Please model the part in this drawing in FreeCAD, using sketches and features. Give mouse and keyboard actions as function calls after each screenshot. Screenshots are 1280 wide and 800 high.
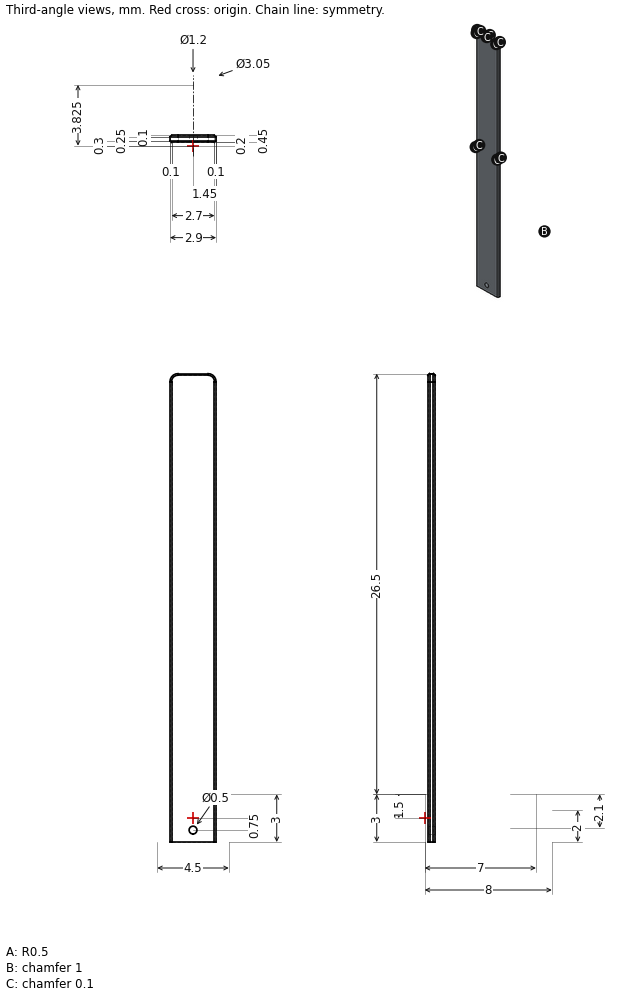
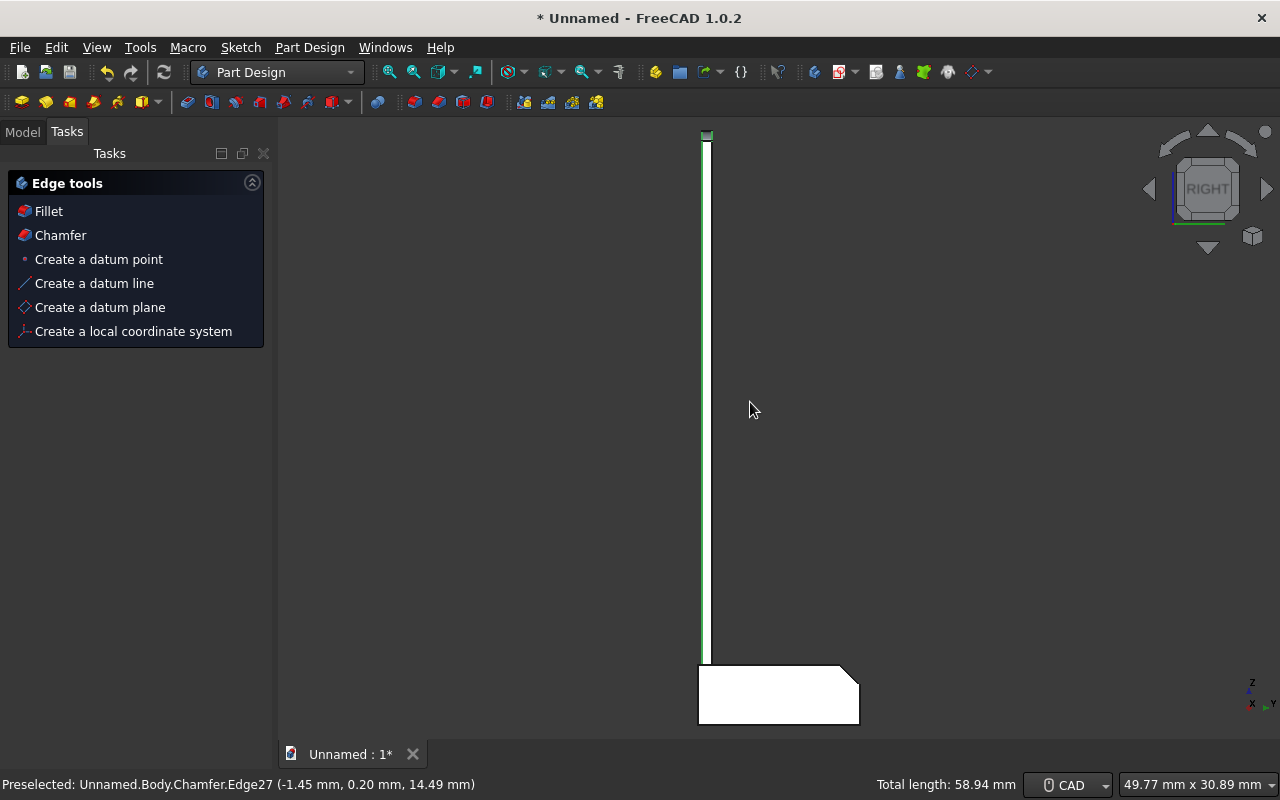
click(712, 402, ctrl)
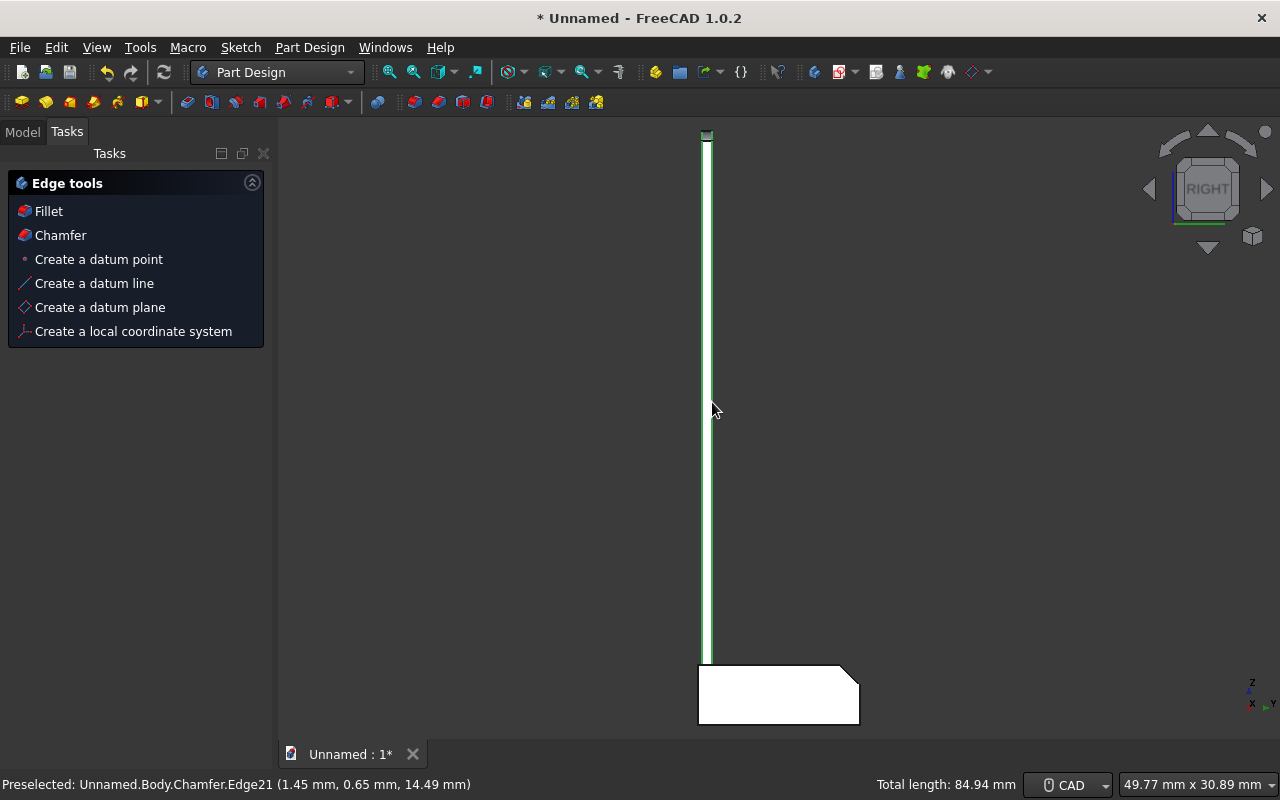
key(5)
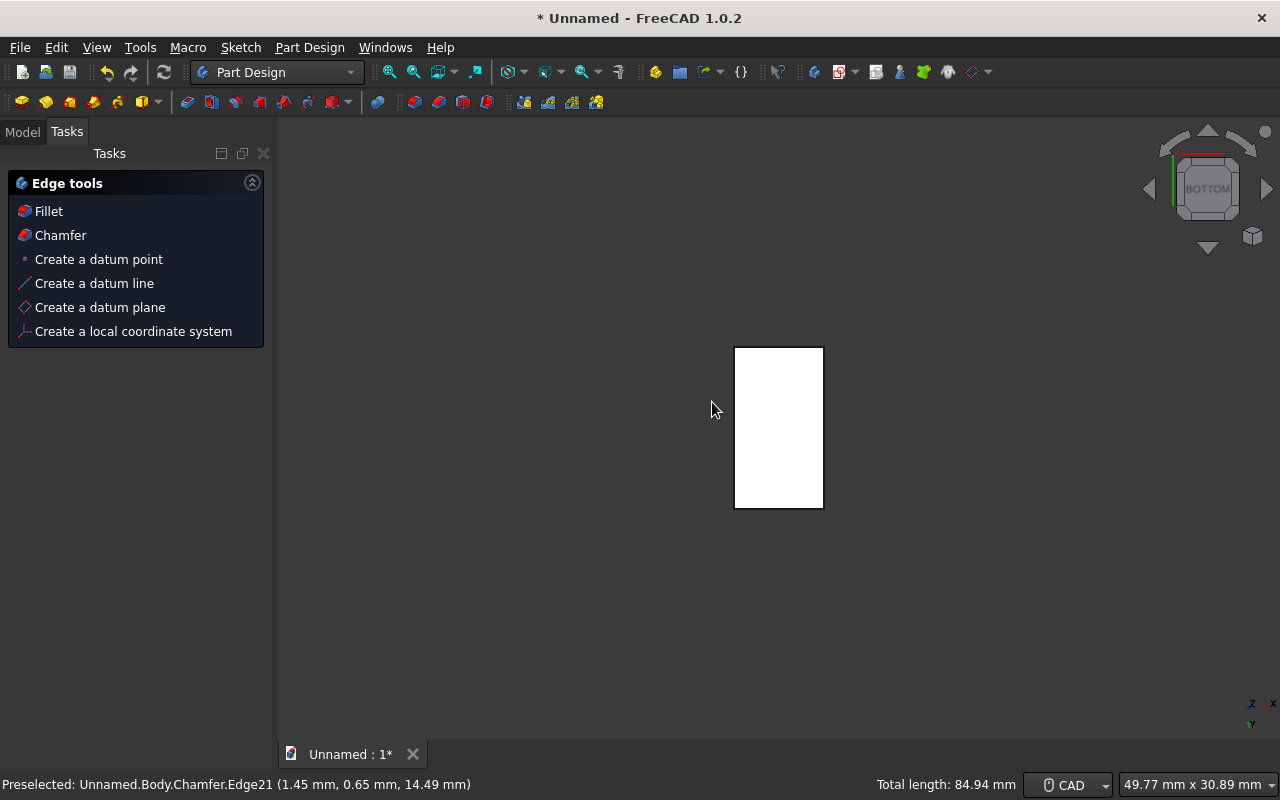
key(v)
key(f)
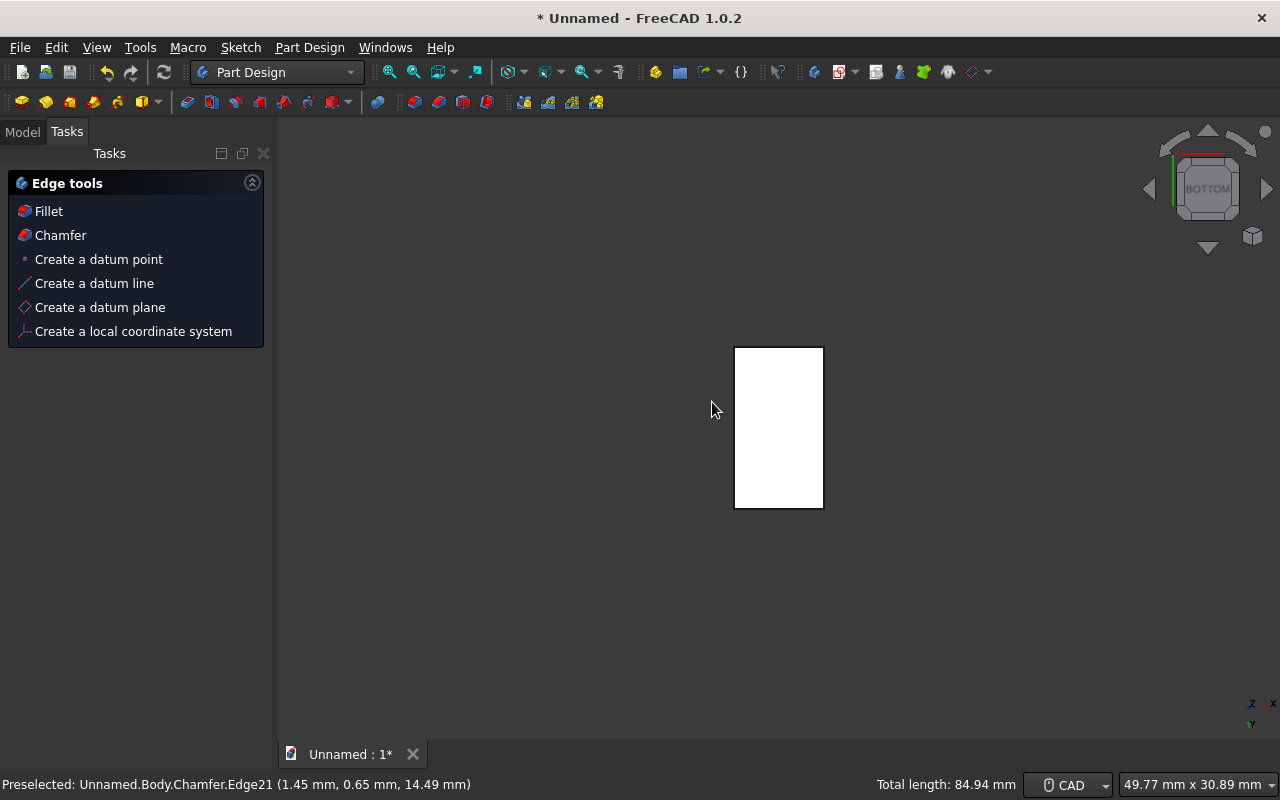
key(4)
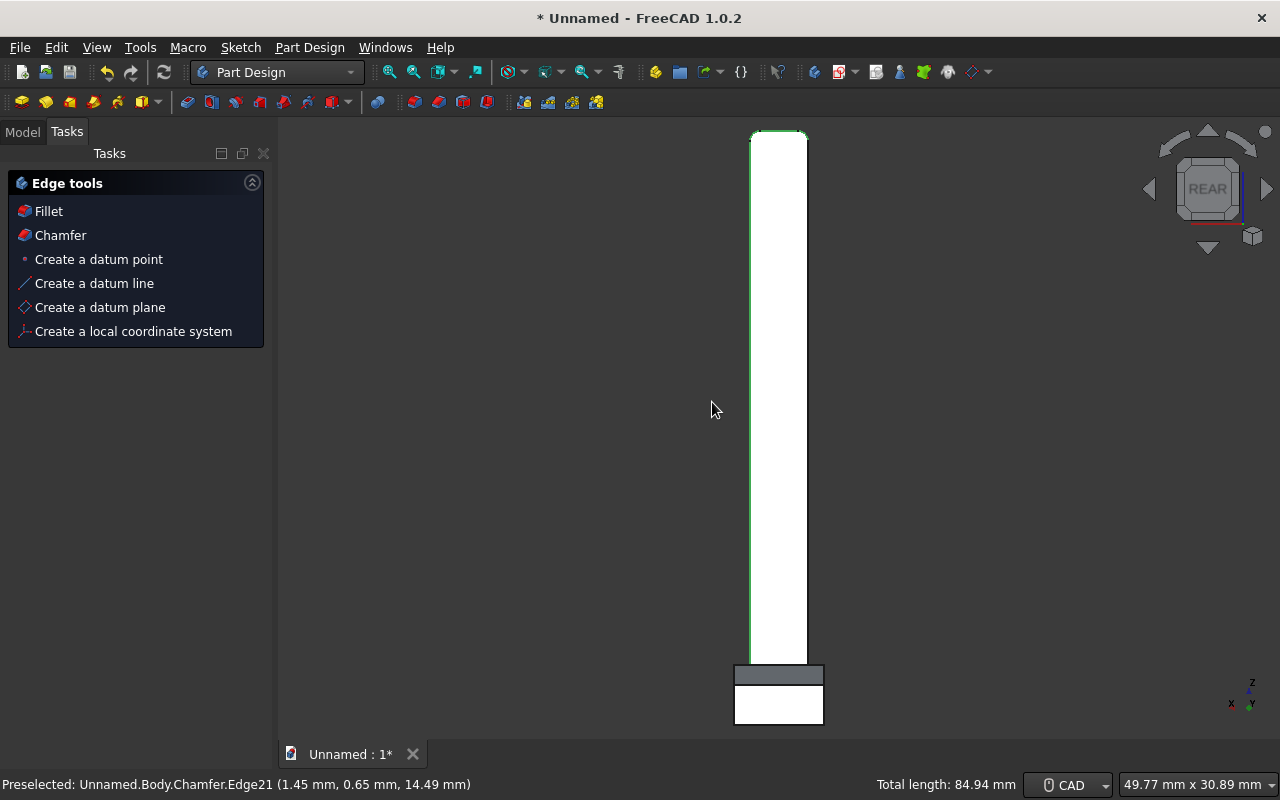
click(808, 402, ctrl)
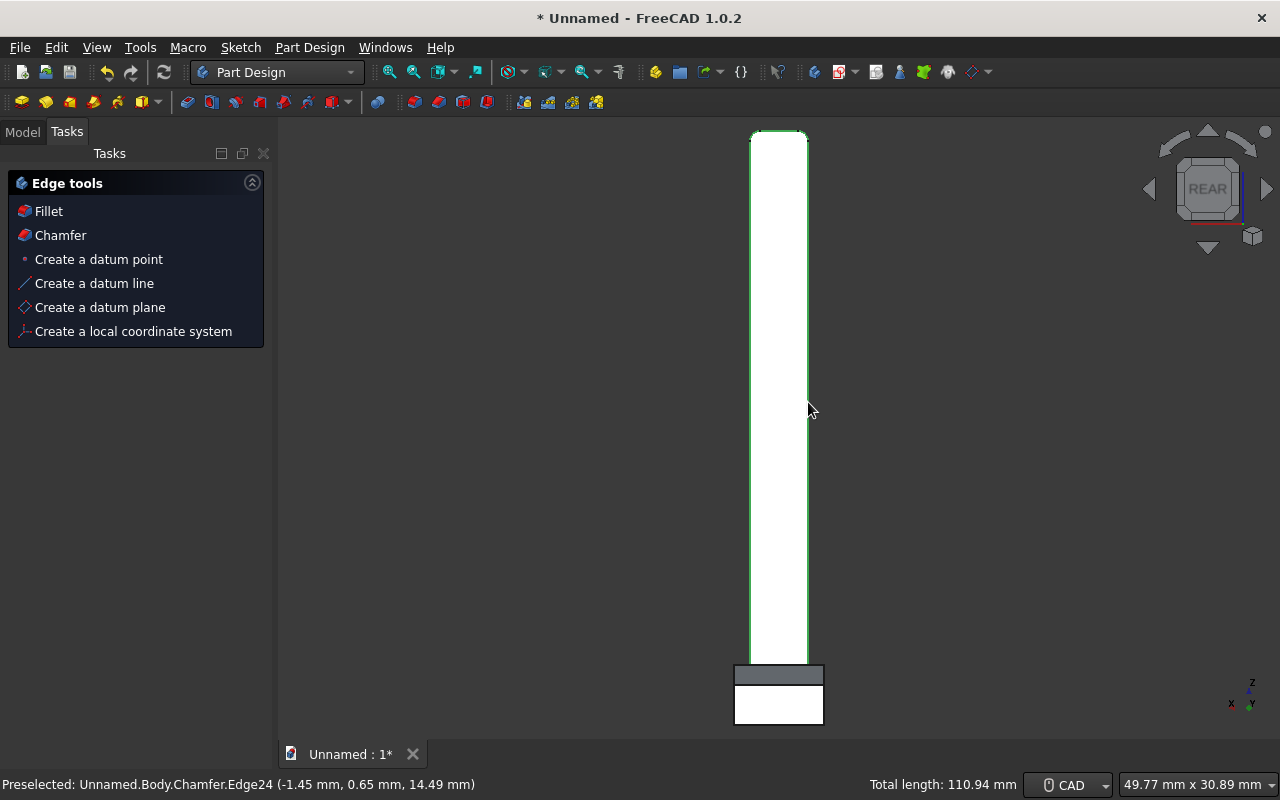
click(440, 102)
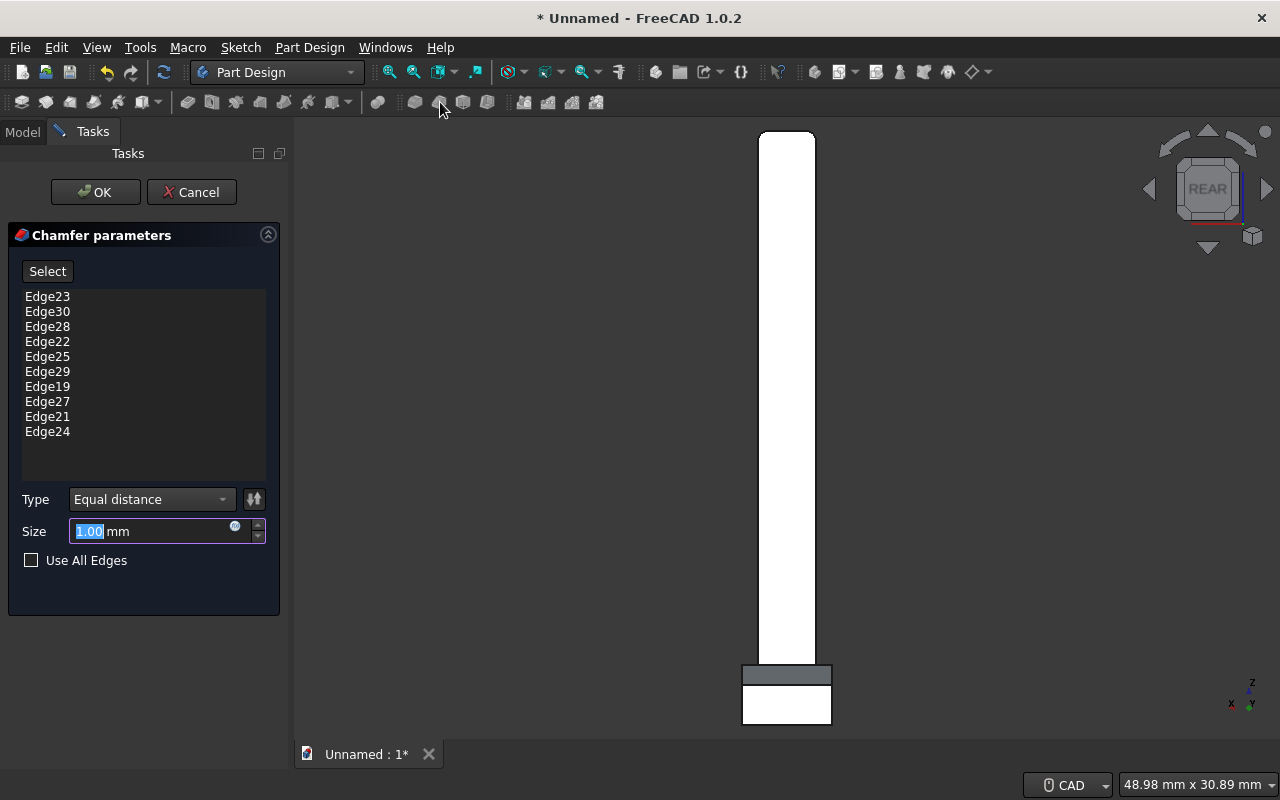
text(0.1)
key(Tab)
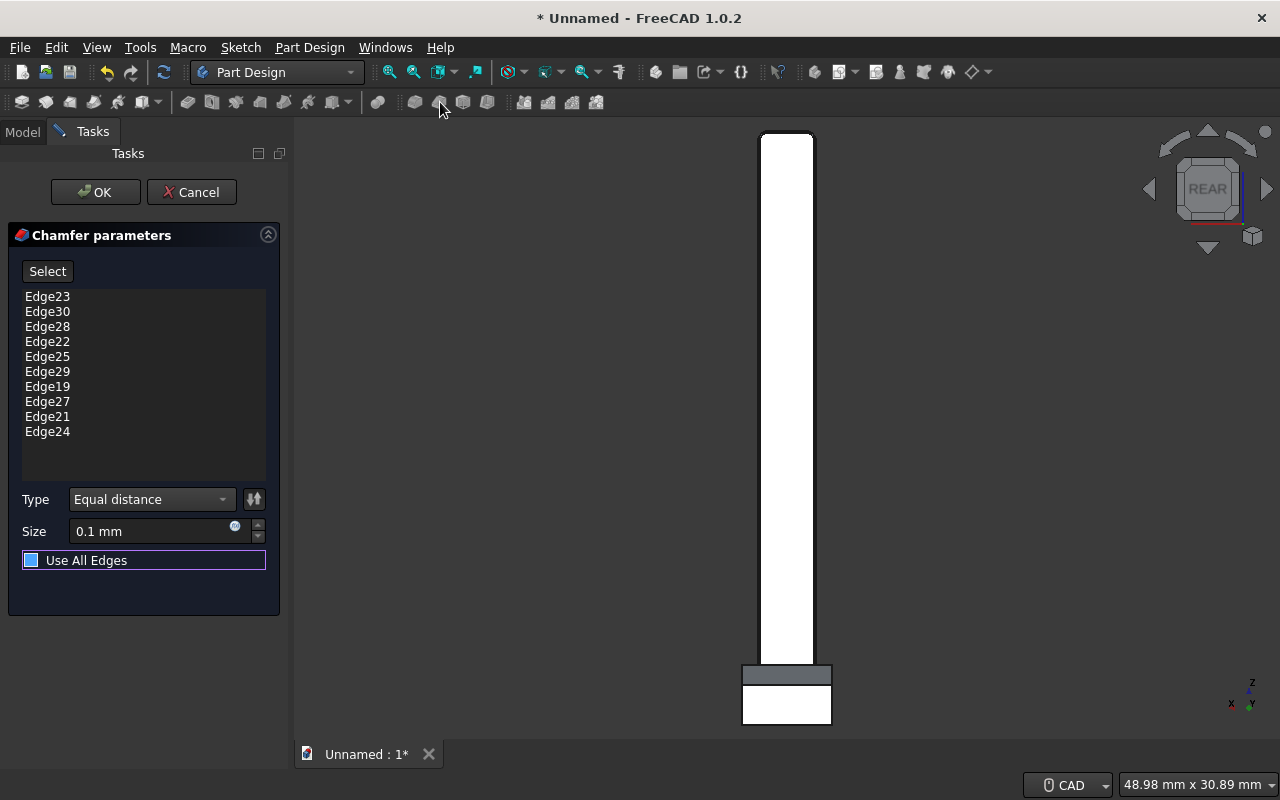
click(96, 192)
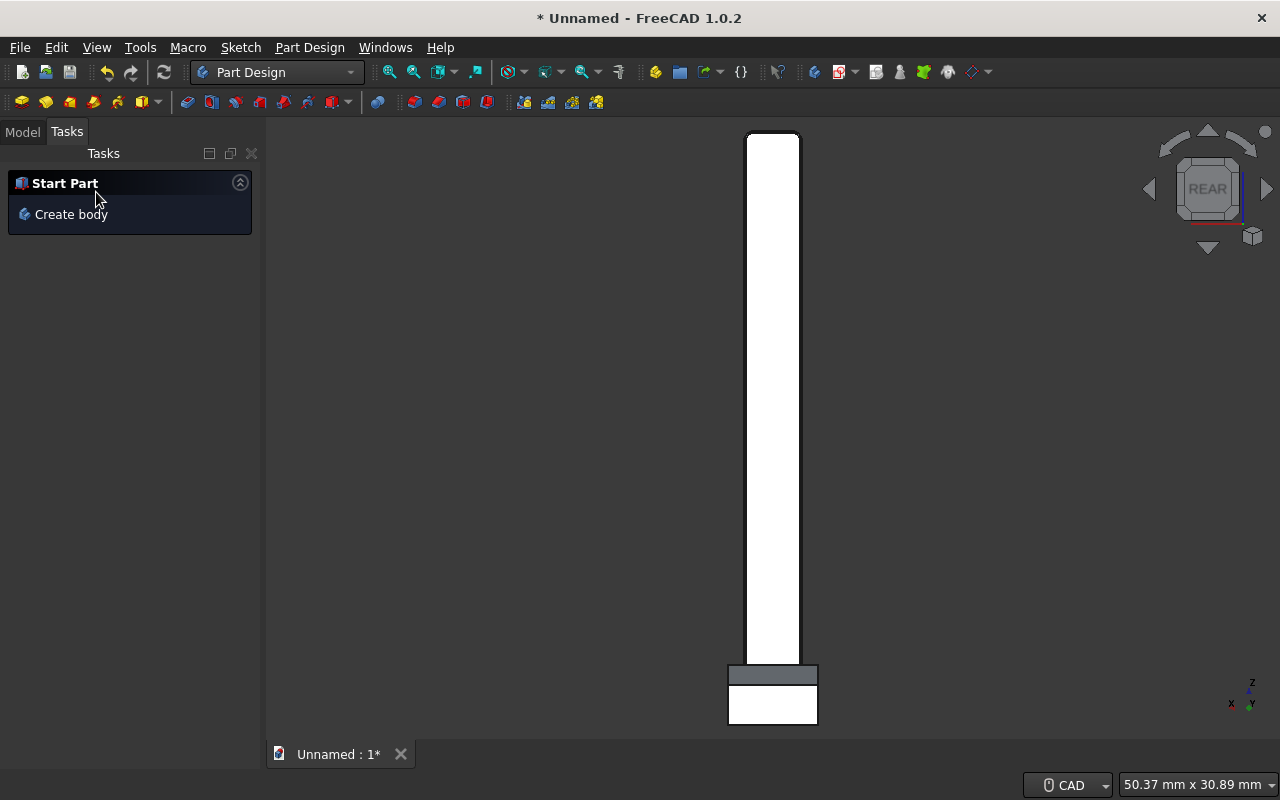
key(0)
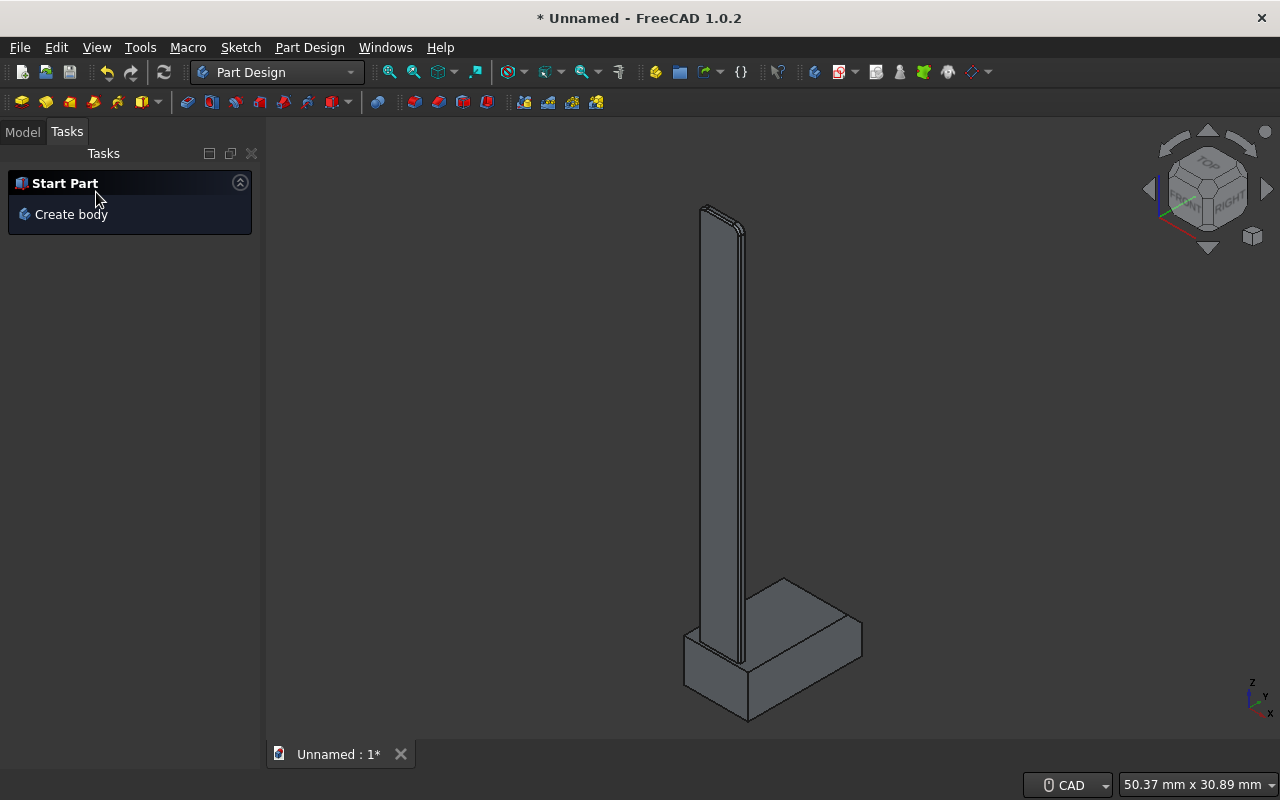
click(780, 616)